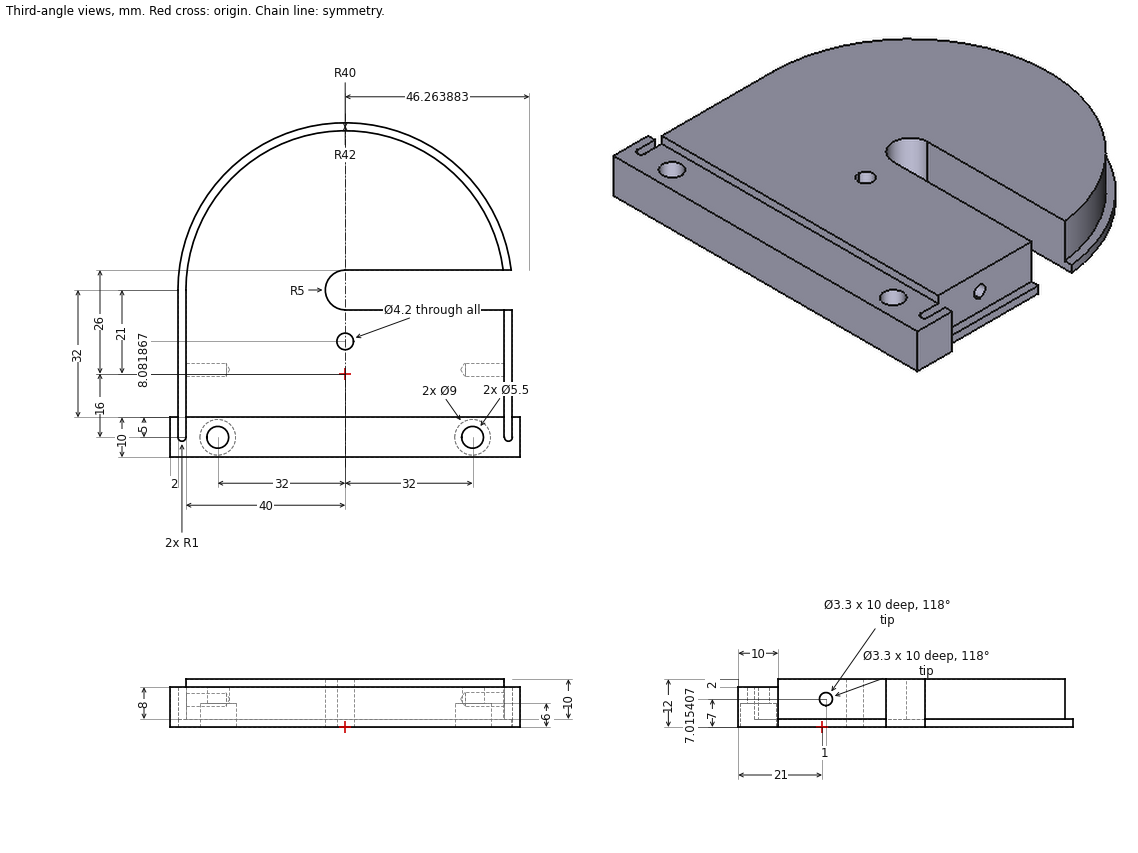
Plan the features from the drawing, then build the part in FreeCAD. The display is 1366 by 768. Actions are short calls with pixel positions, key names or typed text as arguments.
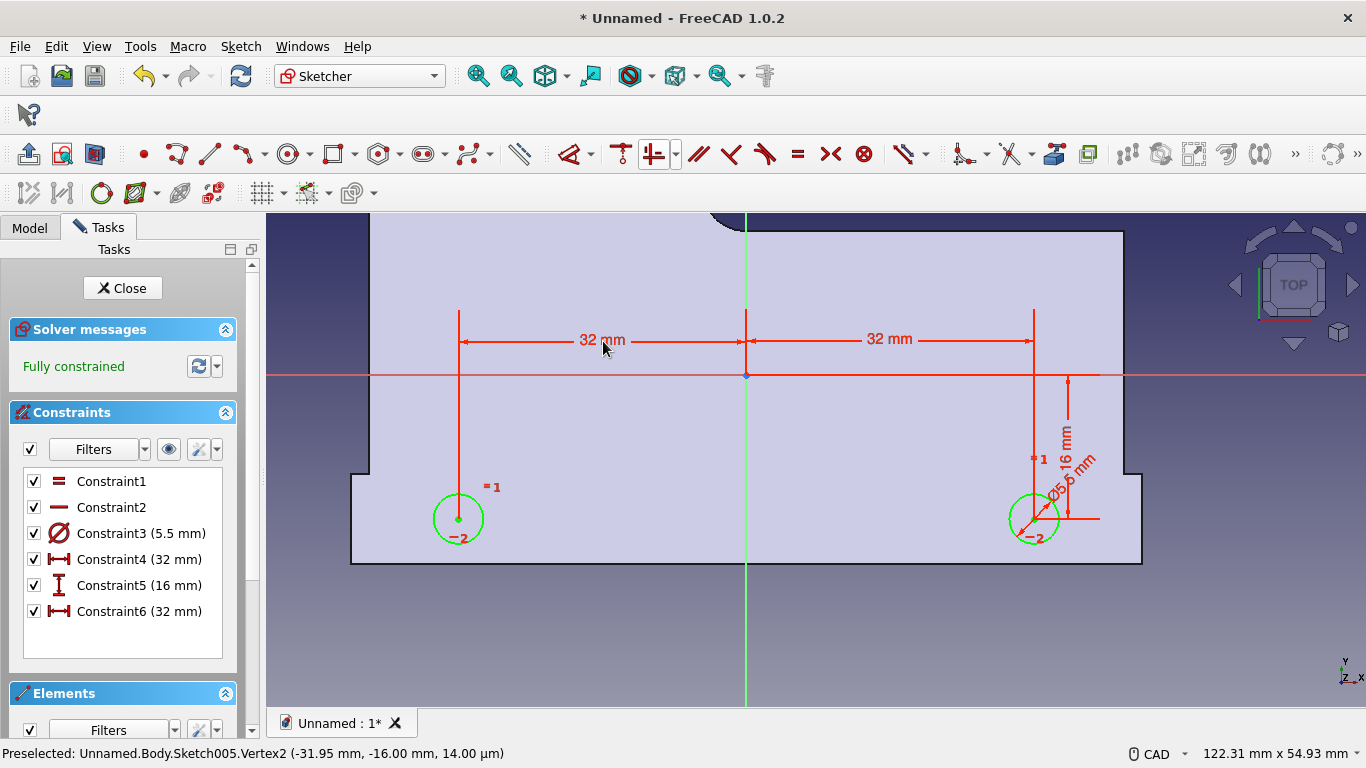
click(123, 288)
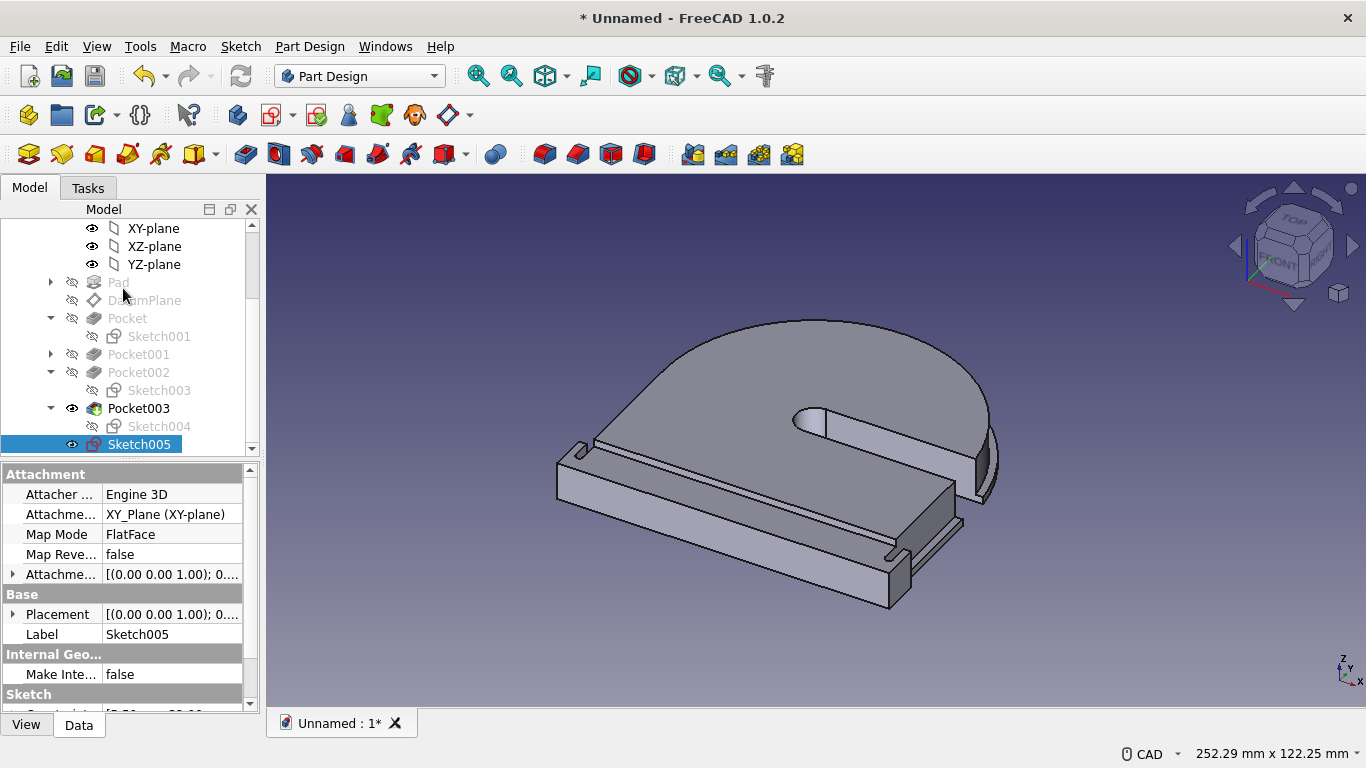
click(246, 154)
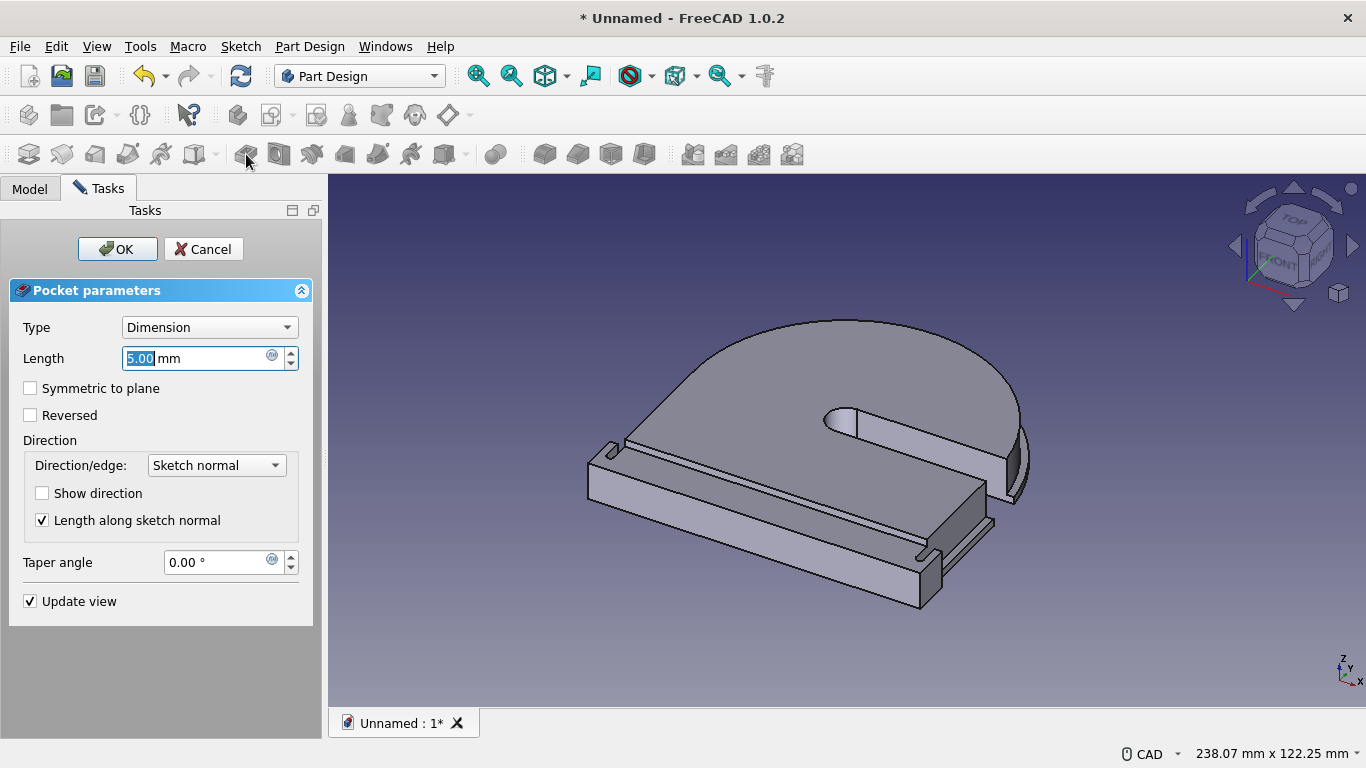
click(210, 328)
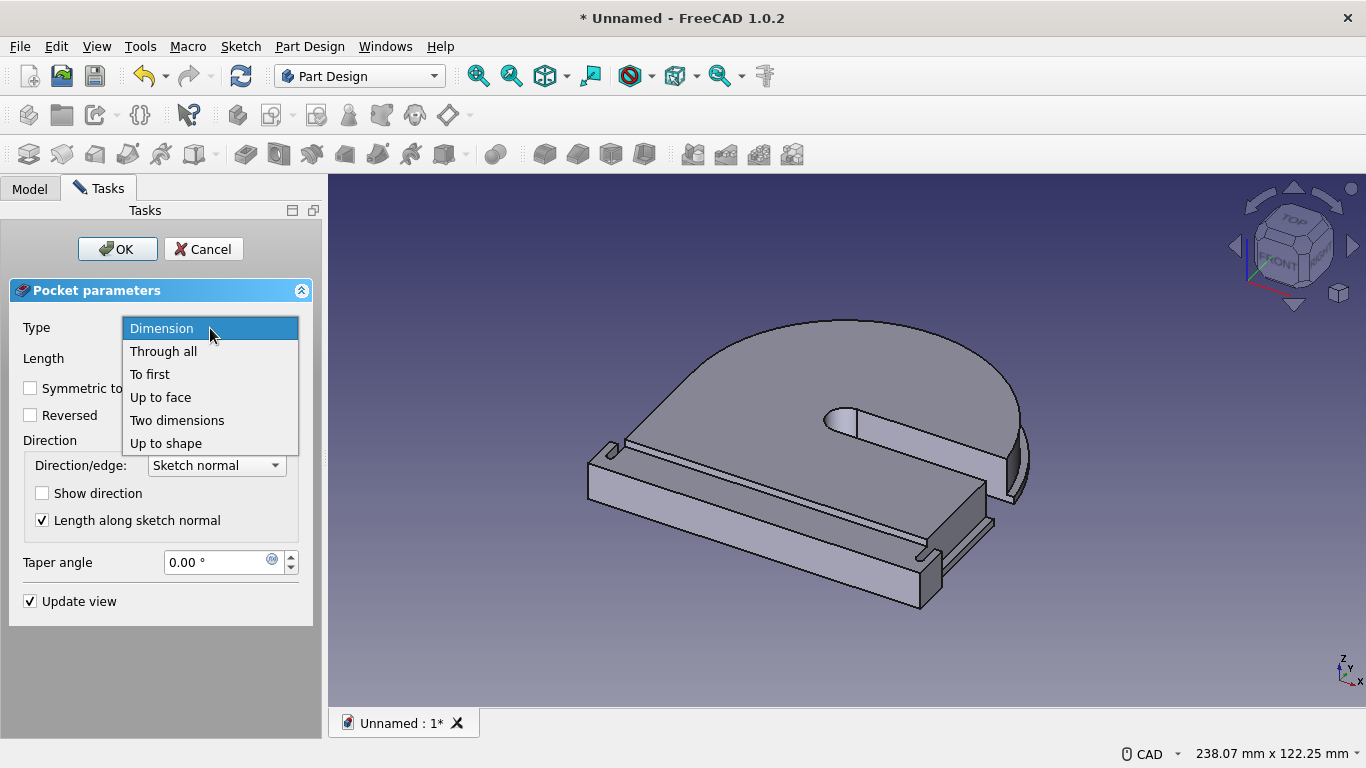
click(208, 352)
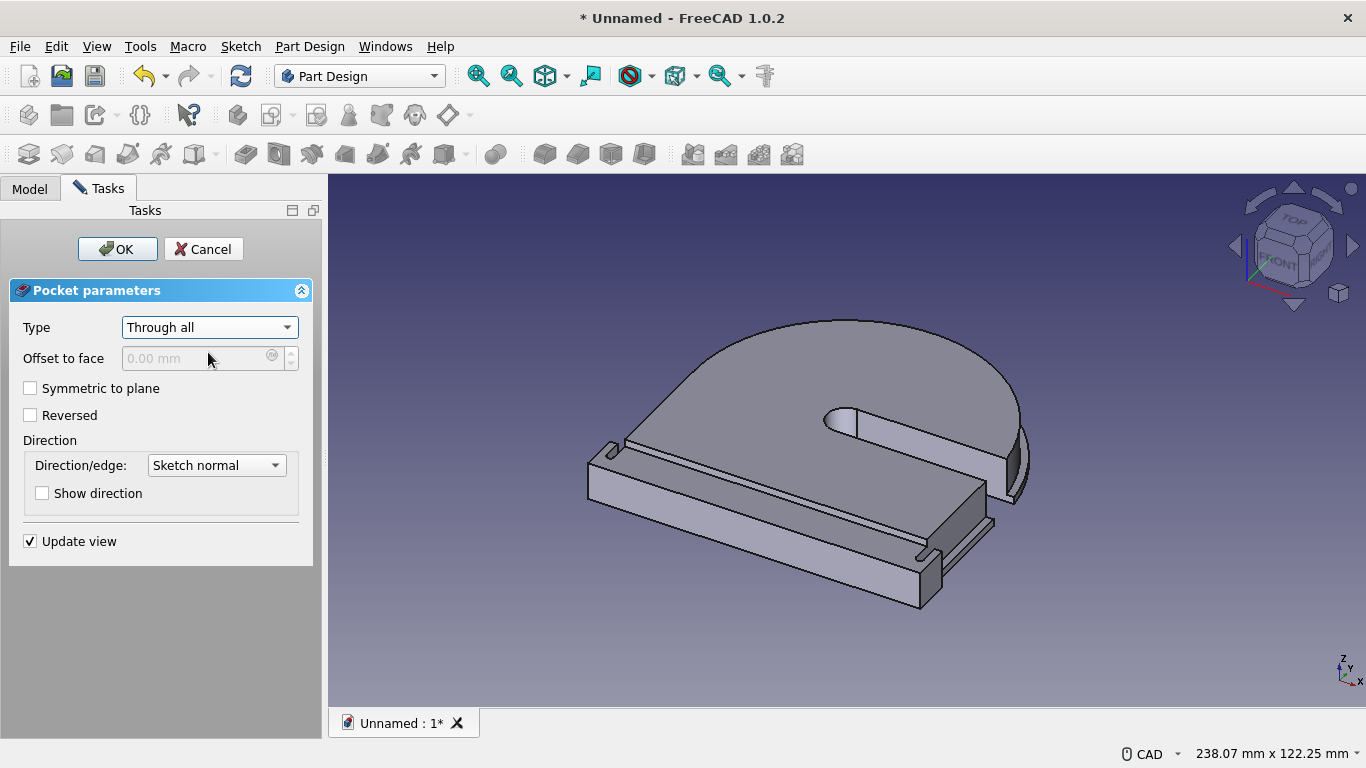
click(31, 415)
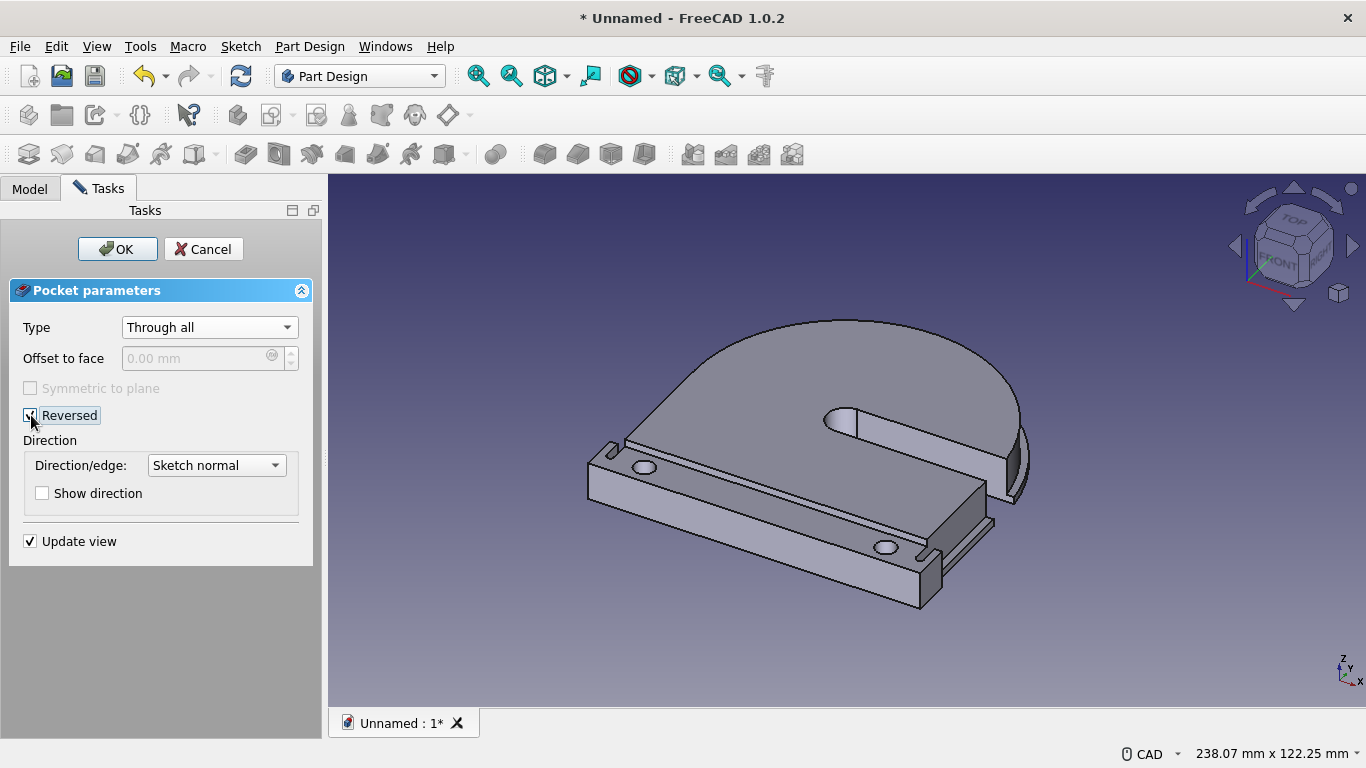
click(118, 249)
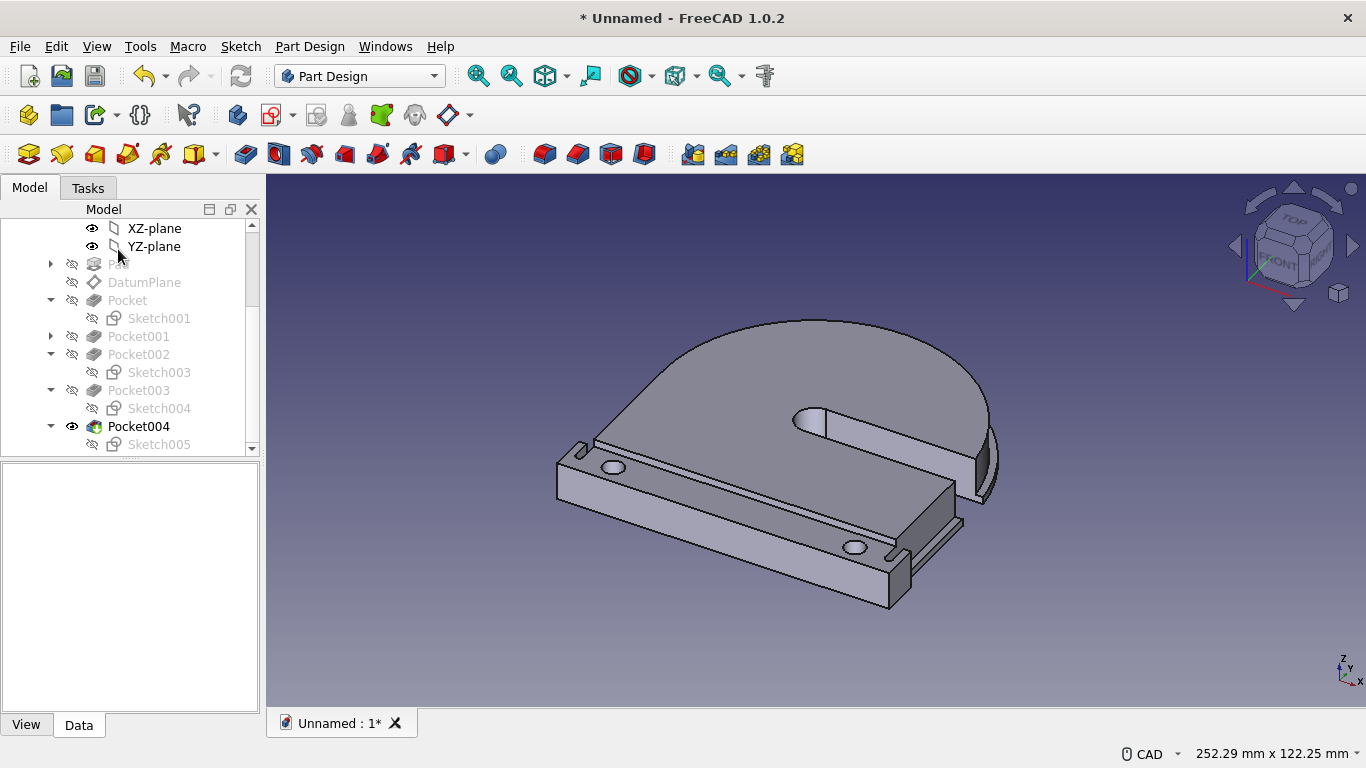
click(270, 116)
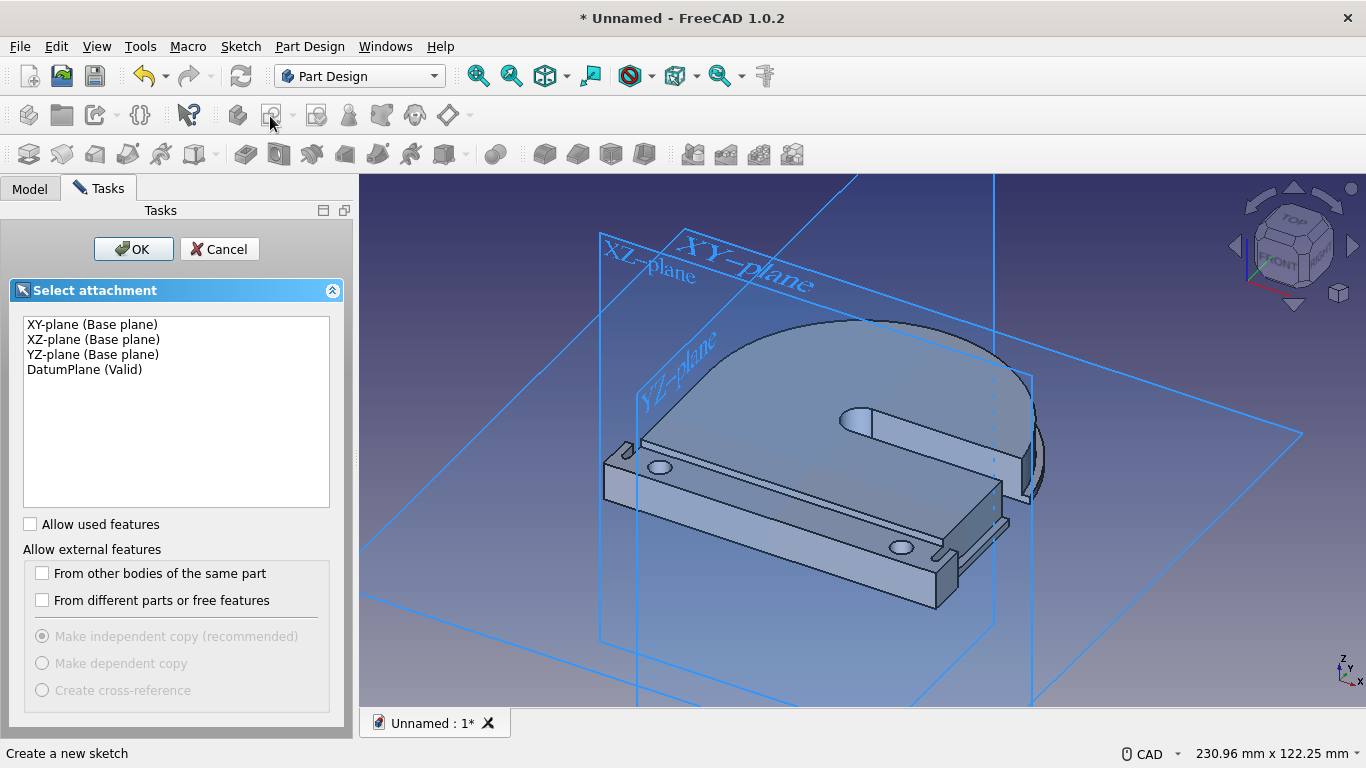
click(84, 324)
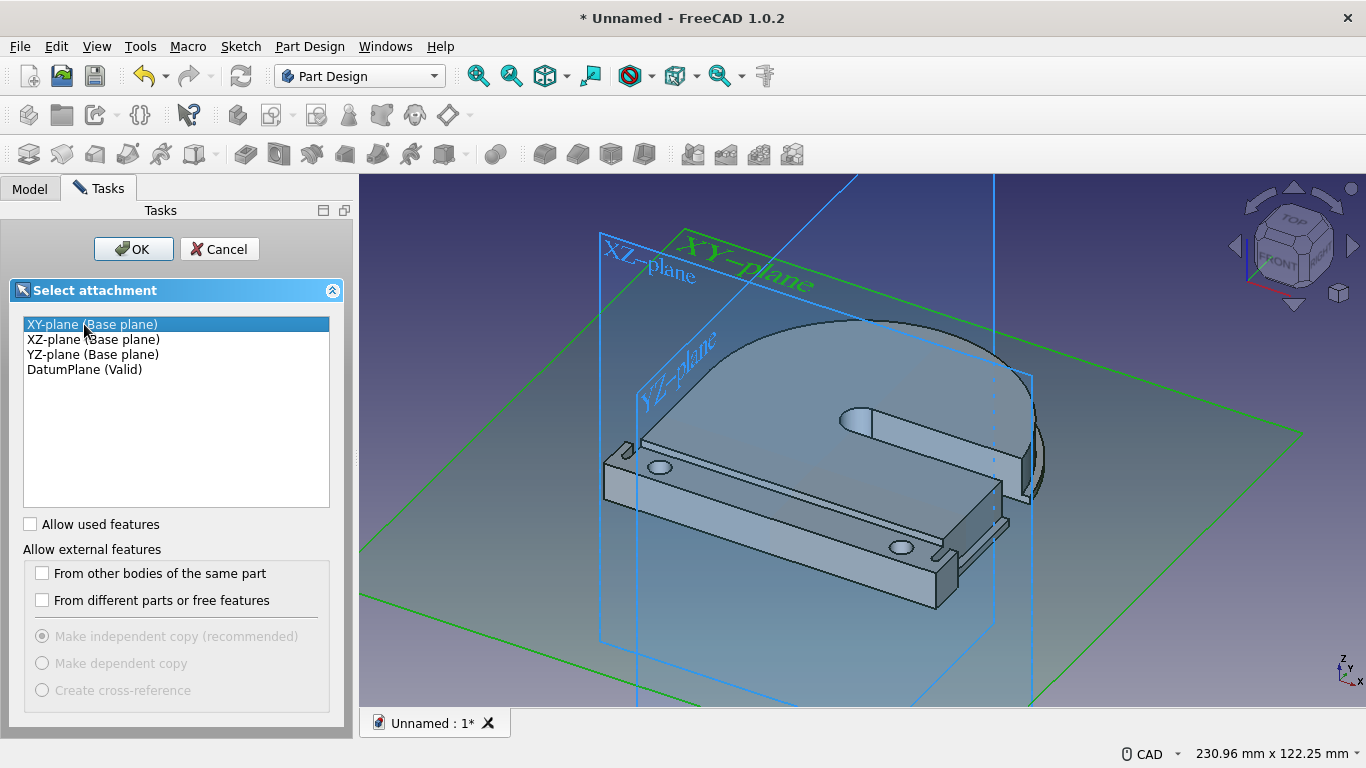
click(134, 249)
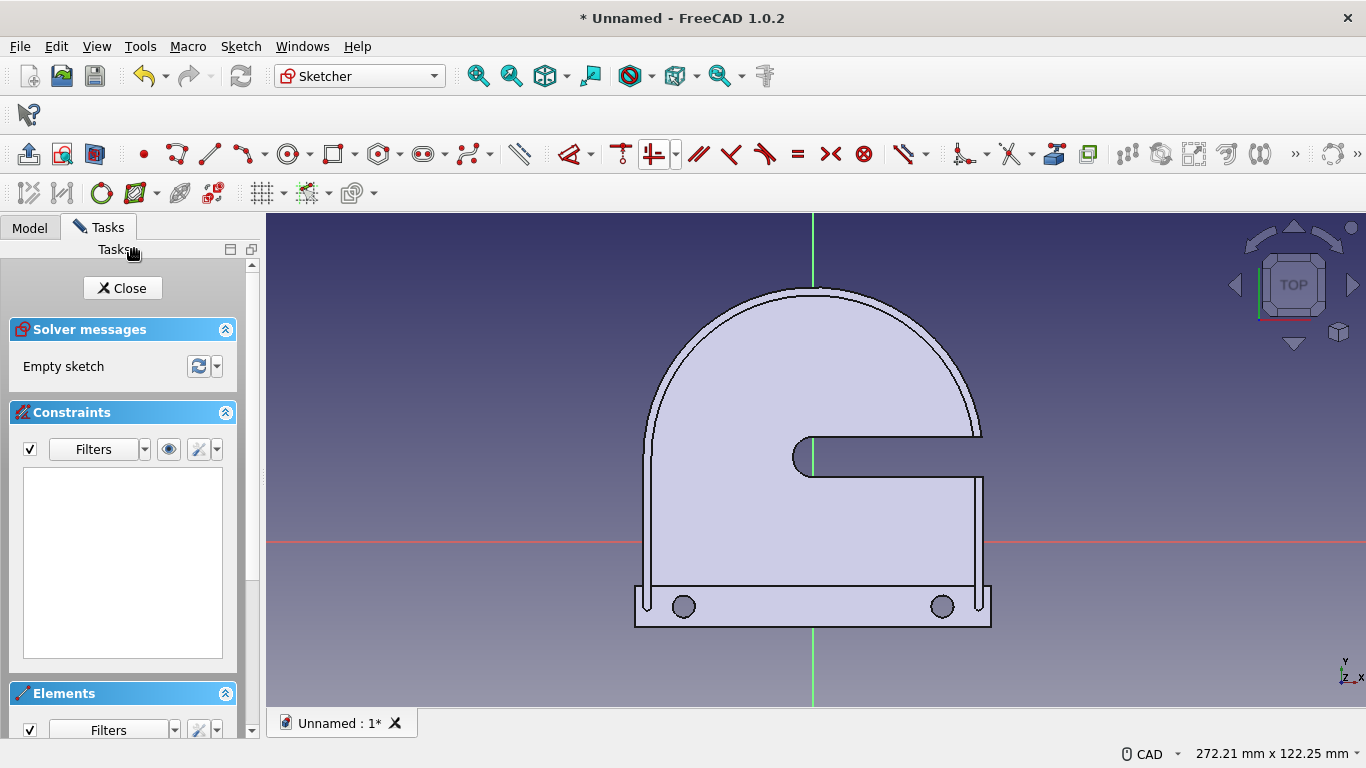
click(95, 154)